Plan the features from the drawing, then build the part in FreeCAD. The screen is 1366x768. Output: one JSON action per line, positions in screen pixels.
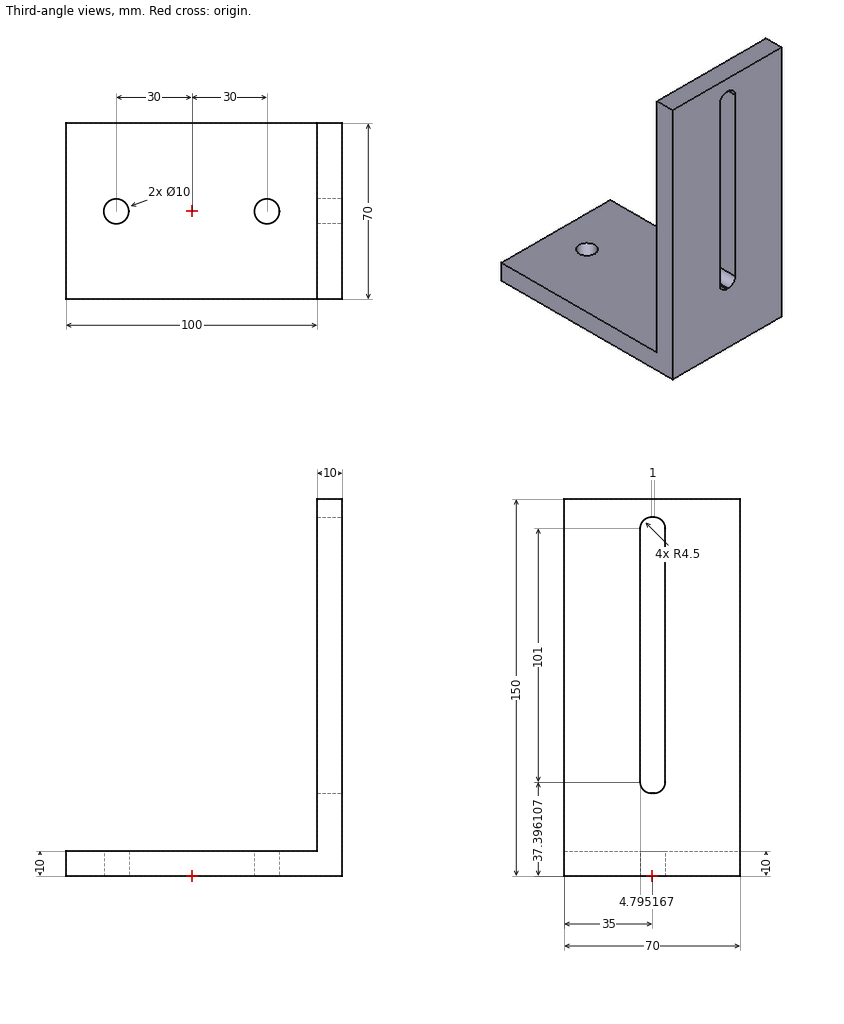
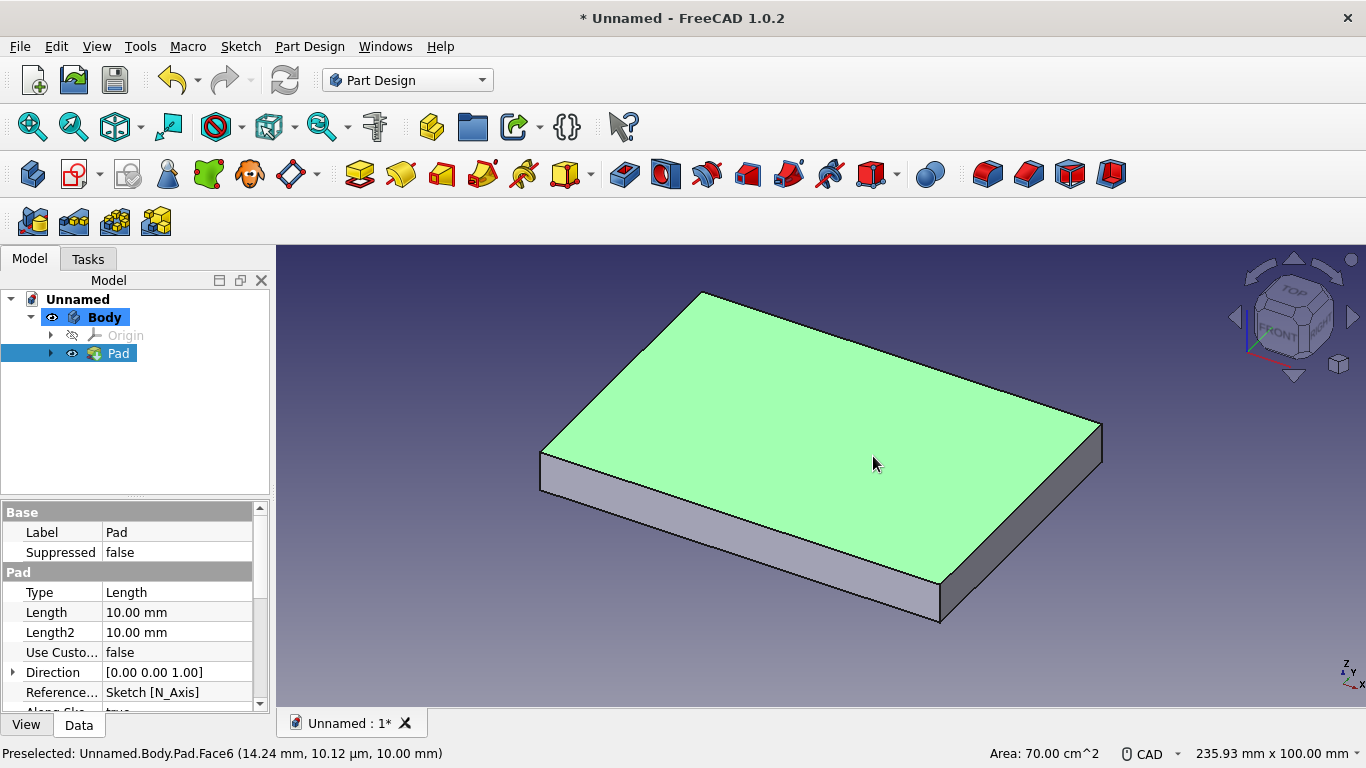
{"action": "left_click", "coordinate": [74, 174]}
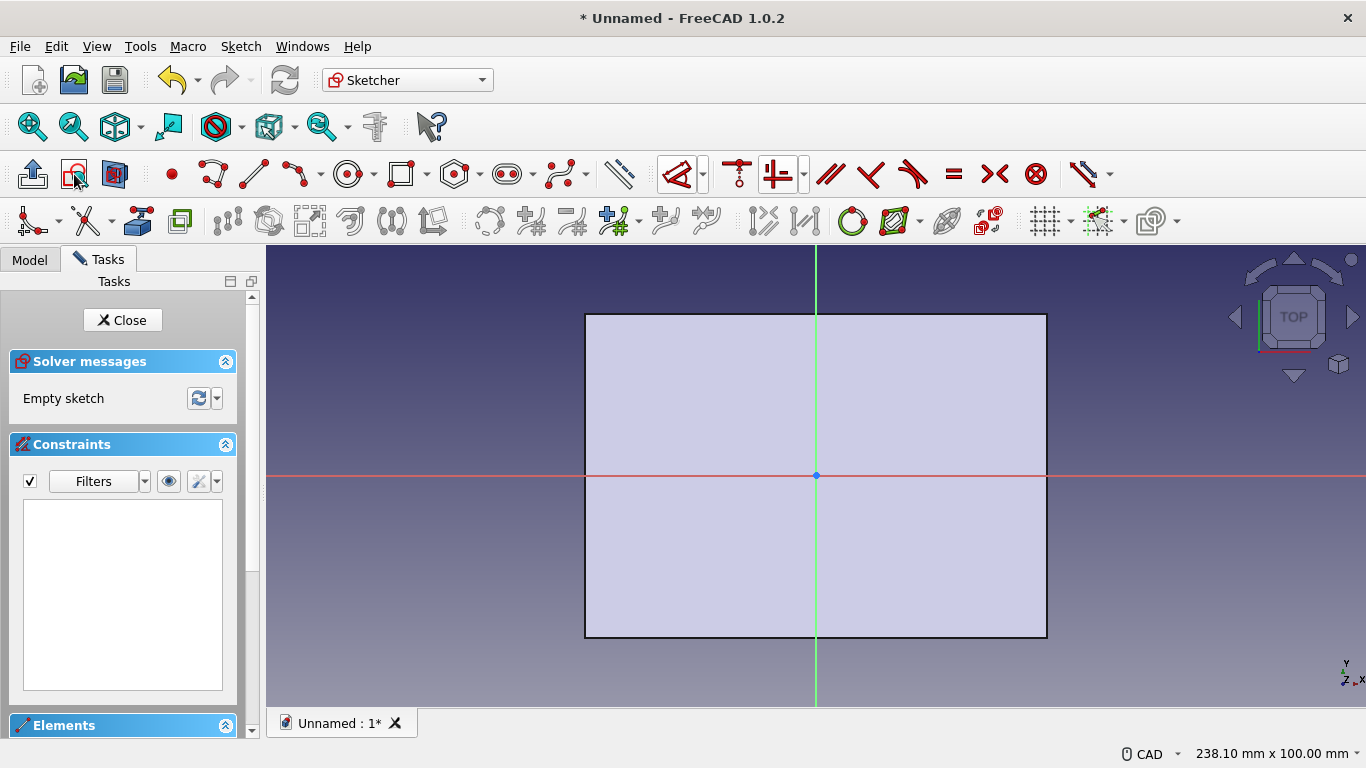
{"action": "scroll", "coordinate": [899, 476], "scroll_direction": "up", "scroll_amount": 3}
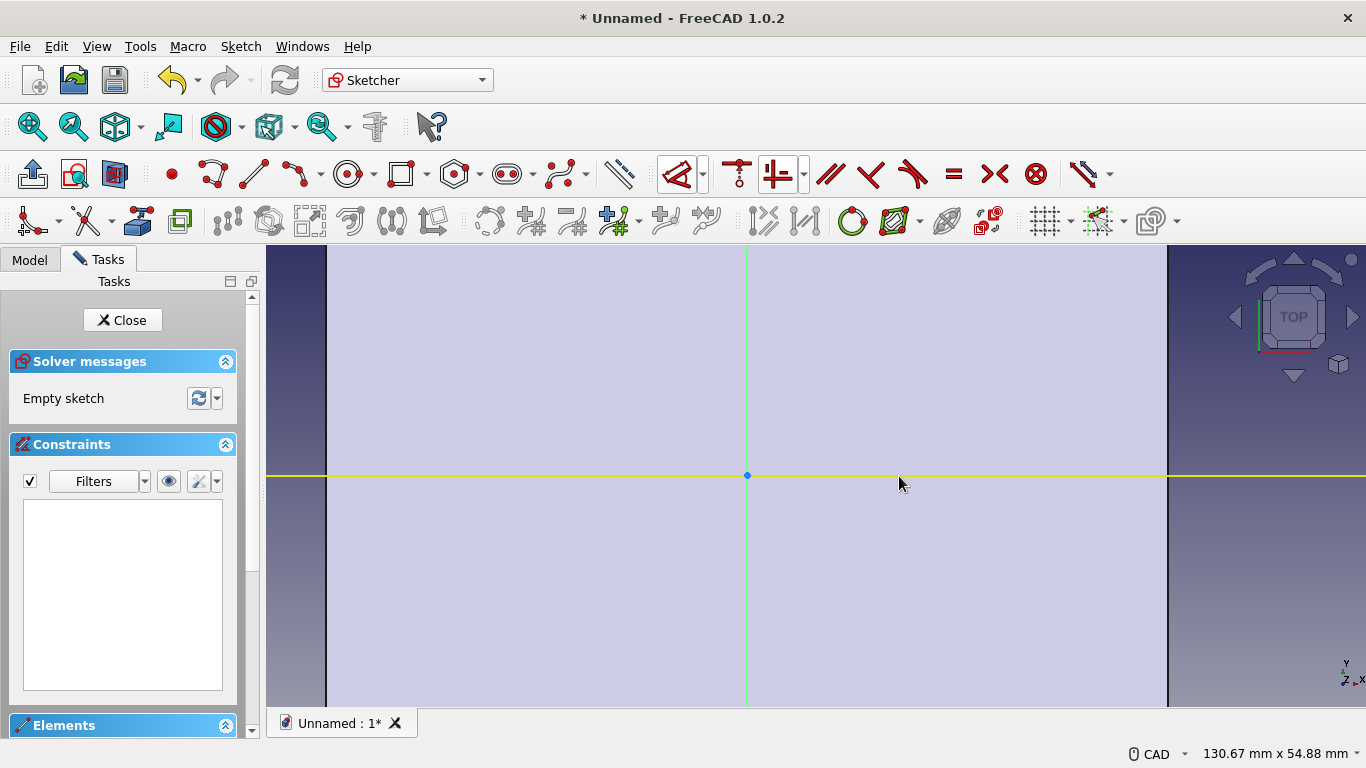
{"action": "left_click", "coordinate": [348, 174]}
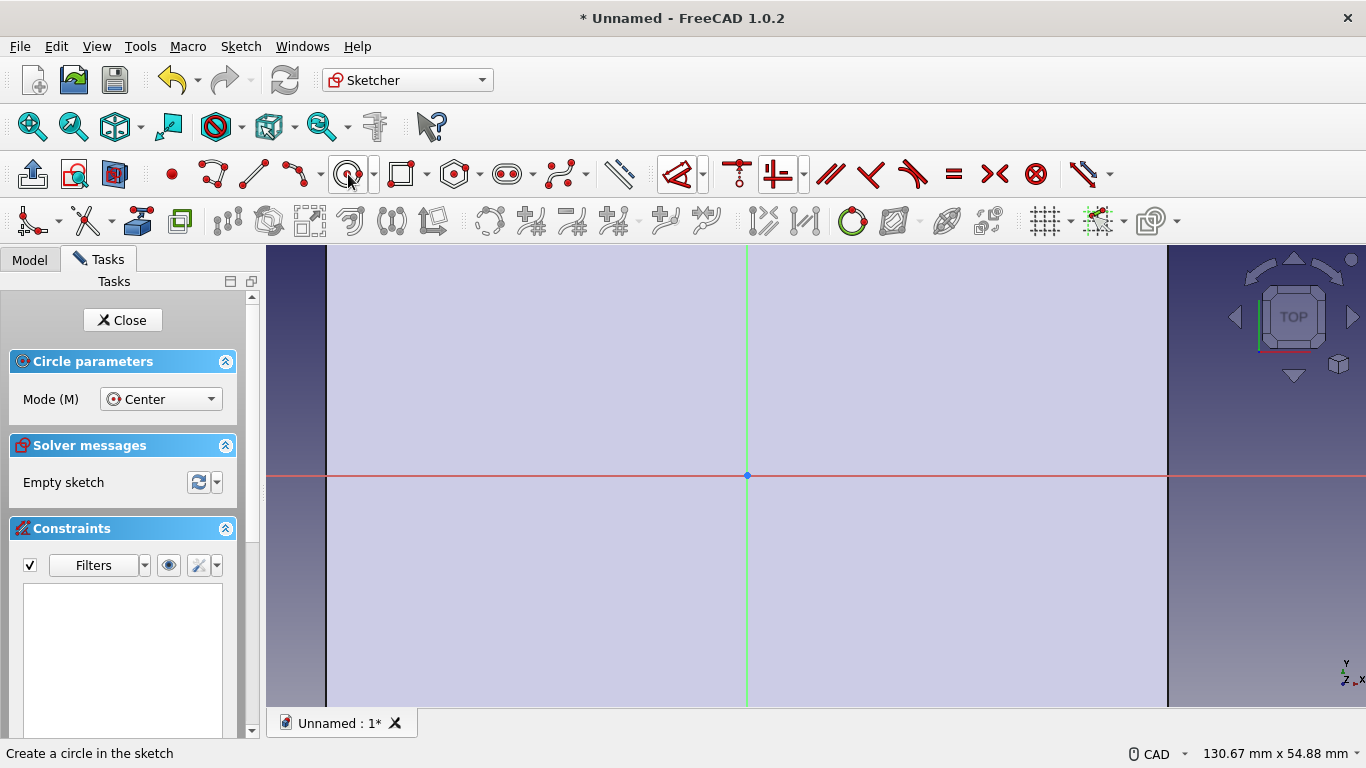
{"action": "left_click", "coordinate": [495, 476]}
{"action": "left_click", "coordinate": [525, 446]}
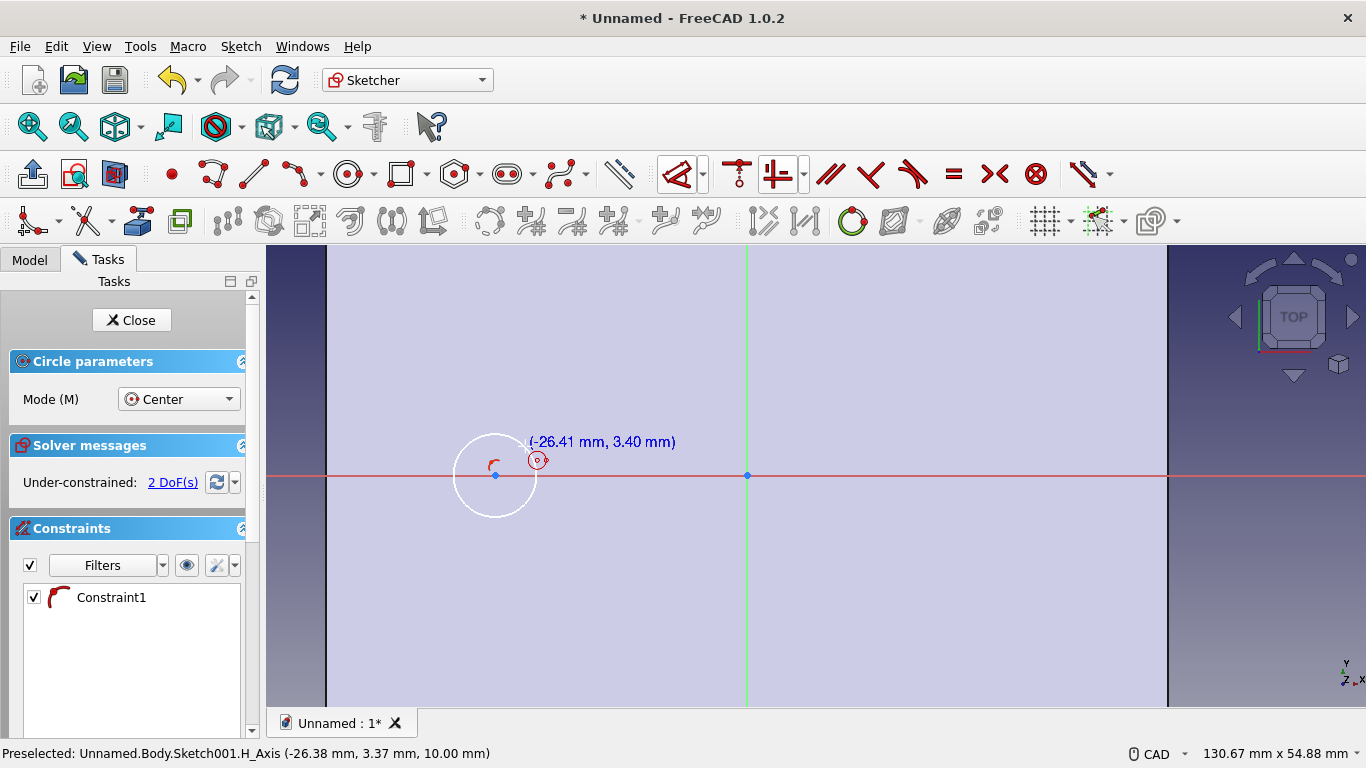
{"action": "left_click", "coordinate": [1000, 476]}
{"action": "left_click", "coordinate": [1030, 446]}
{"action": "key", "text": "Escape"}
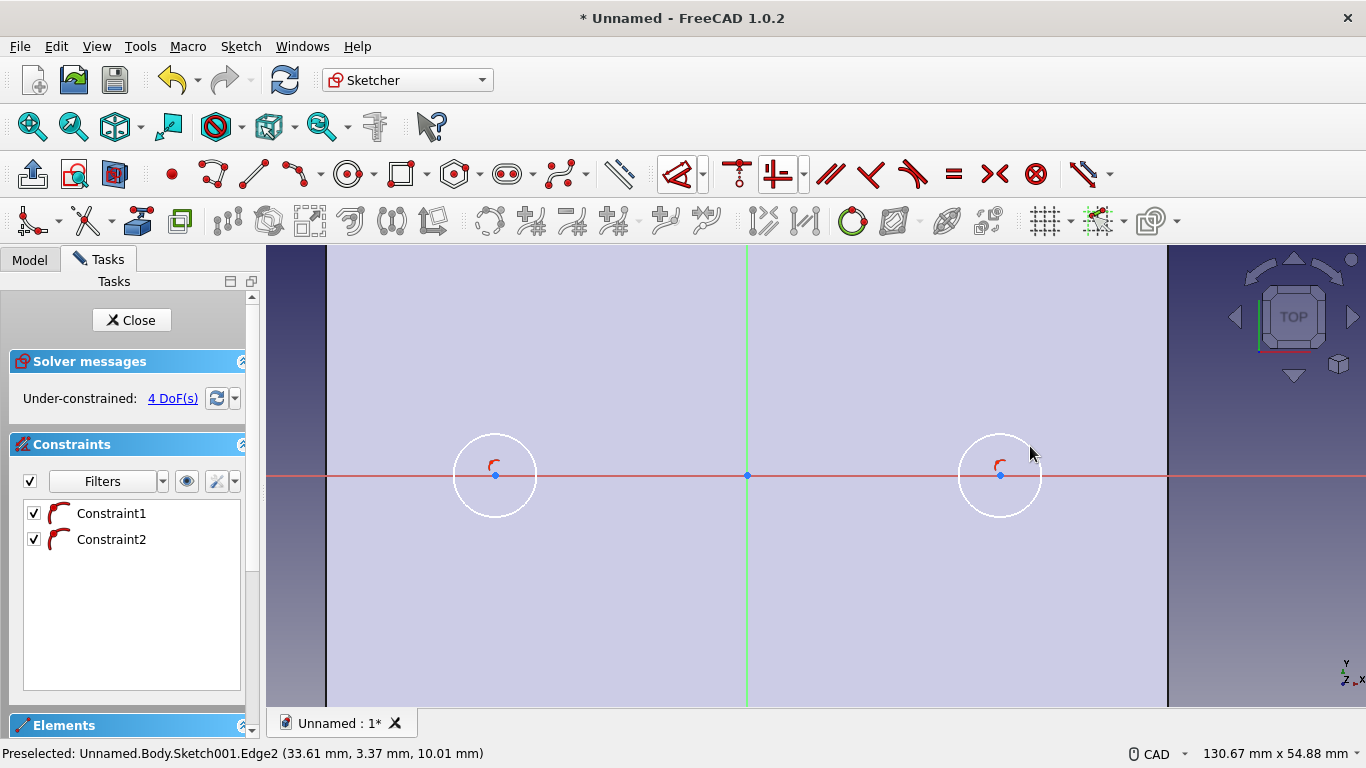
{"action": "left_click", "coordinate": [524, 446]}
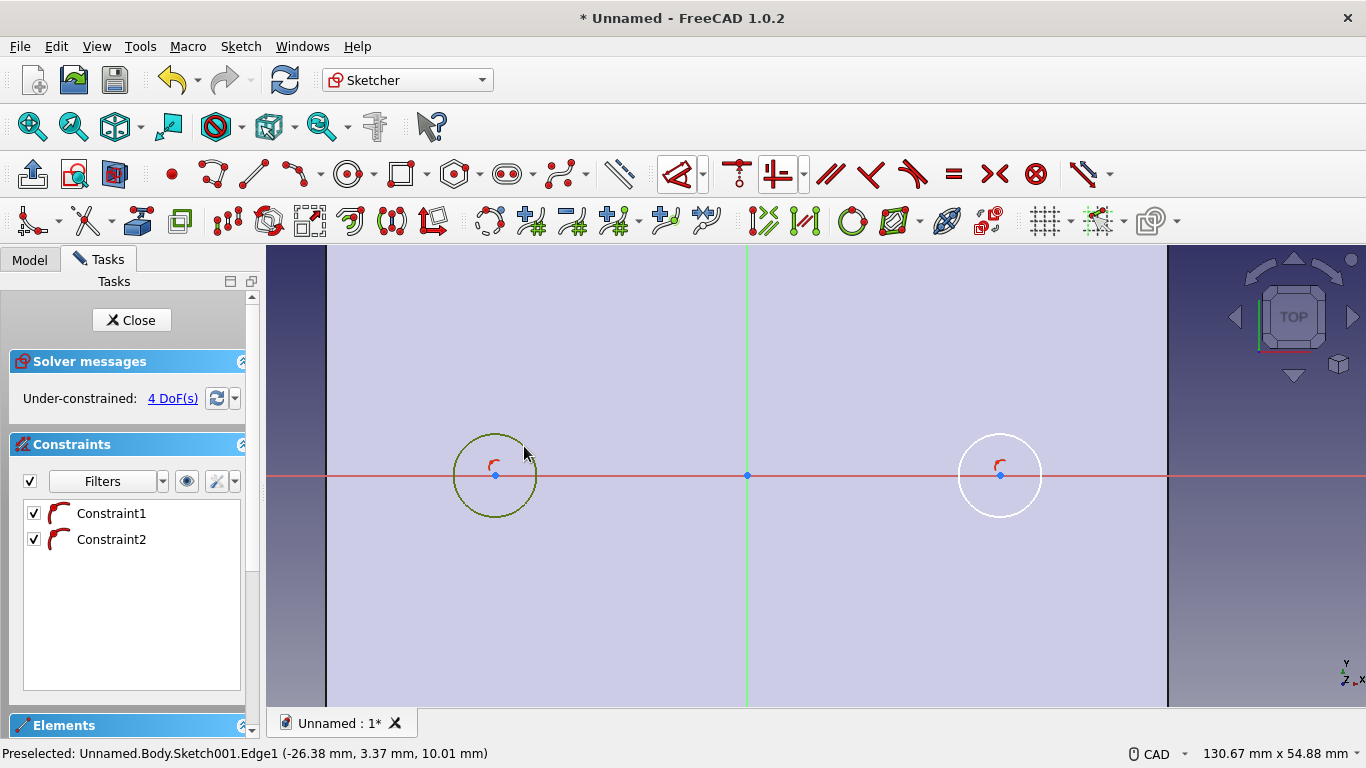
{"action": "left_click", "coordinate": [1029, 446]}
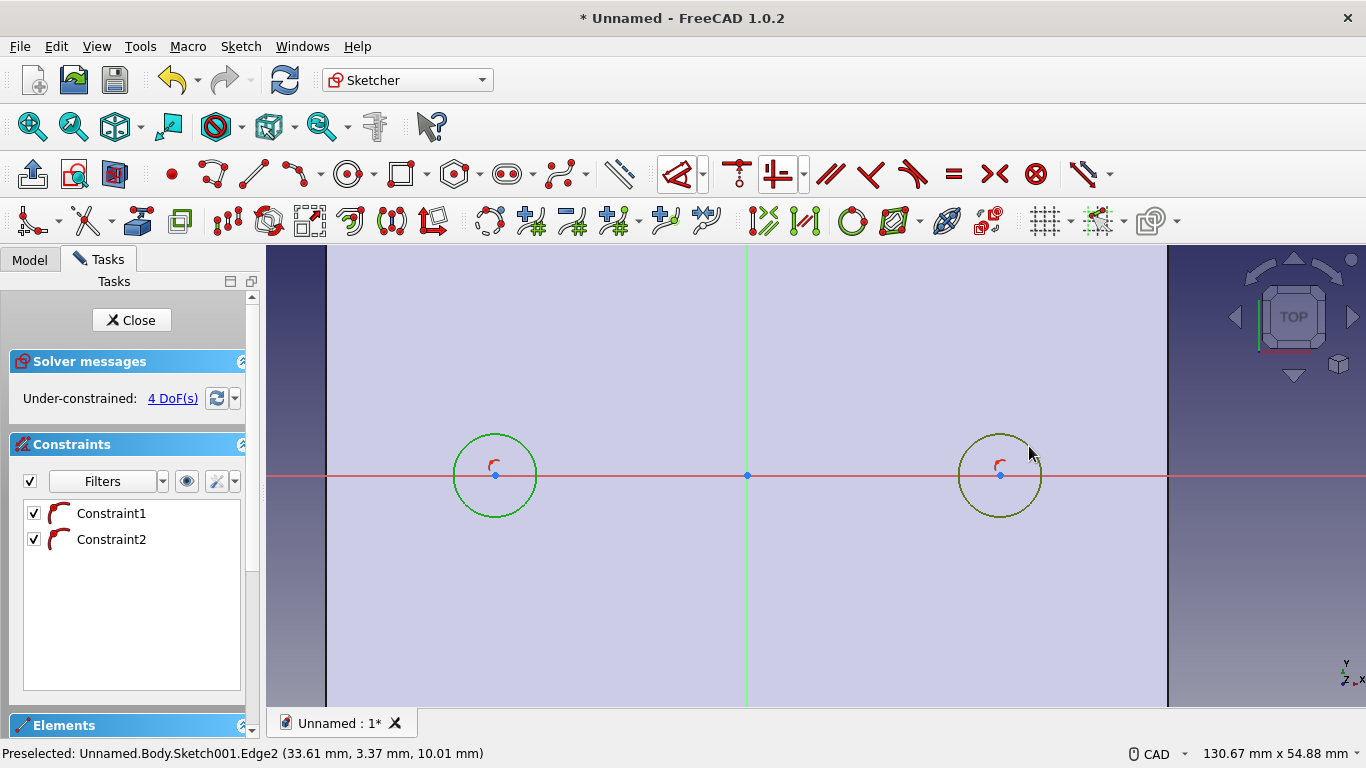
{"action": "left_click", "coordinate": [954, 174]}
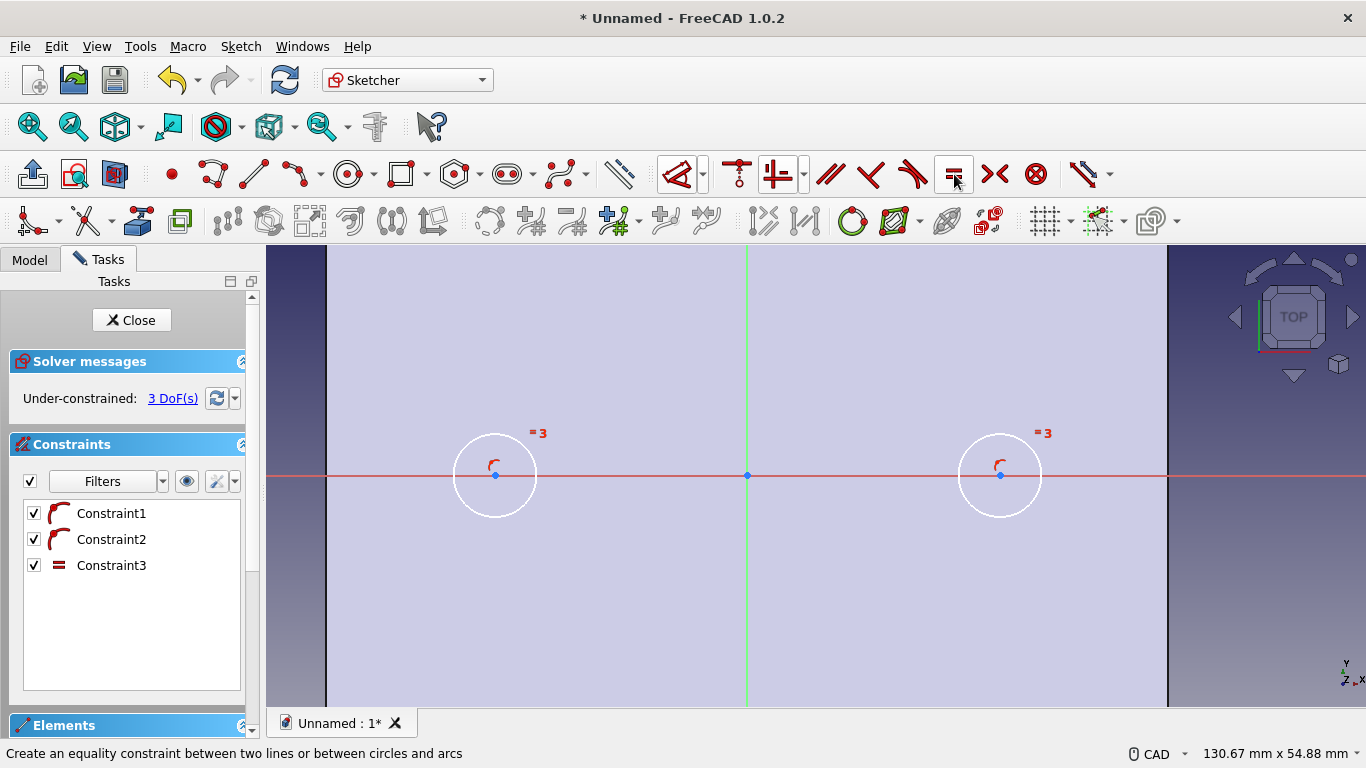
{"action": "left_click", "coordinate": [524, 446]}